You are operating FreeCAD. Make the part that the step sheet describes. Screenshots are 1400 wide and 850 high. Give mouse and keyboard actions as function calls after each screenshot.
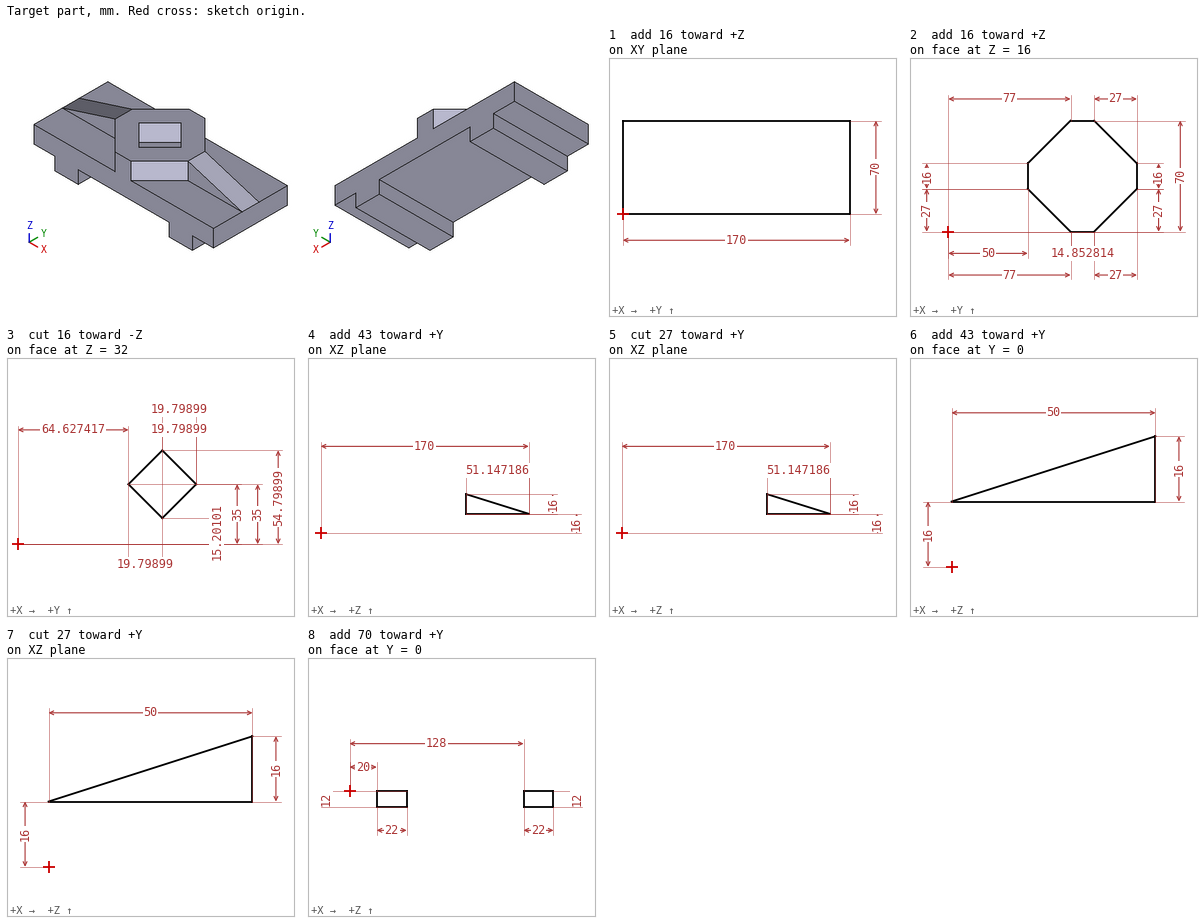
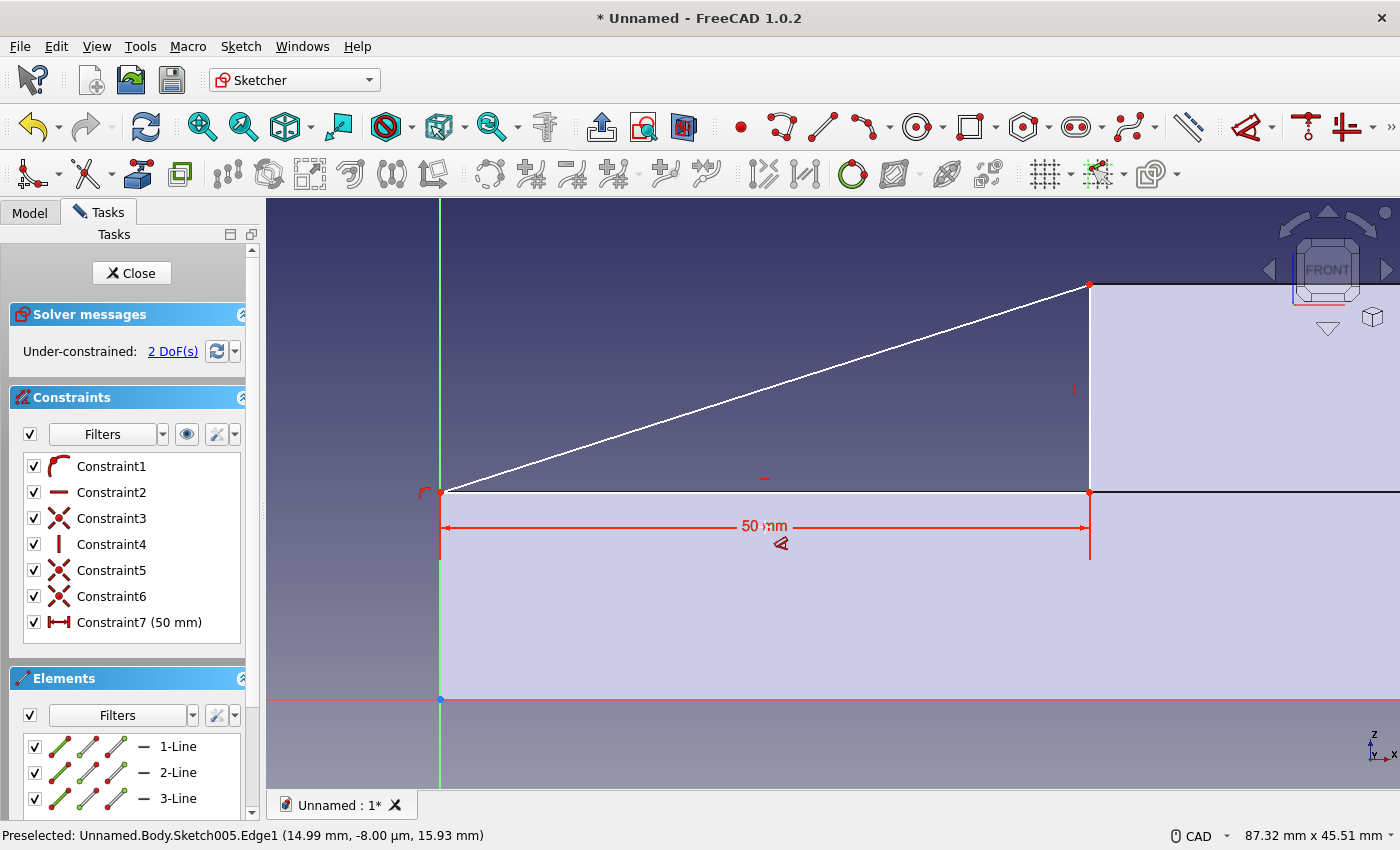
click(1090, 431)
click(1124, 389)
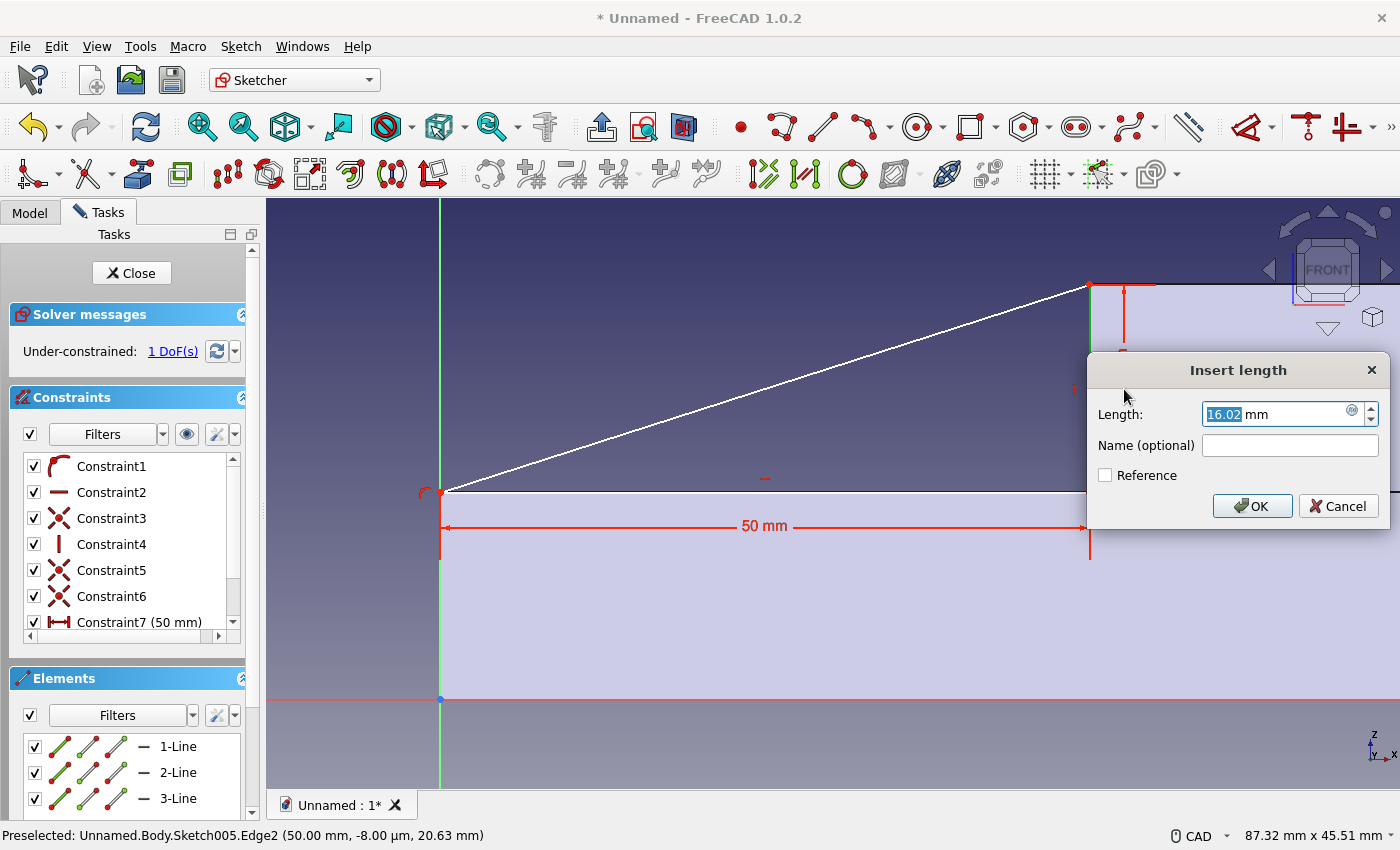
text(16)
key(Return)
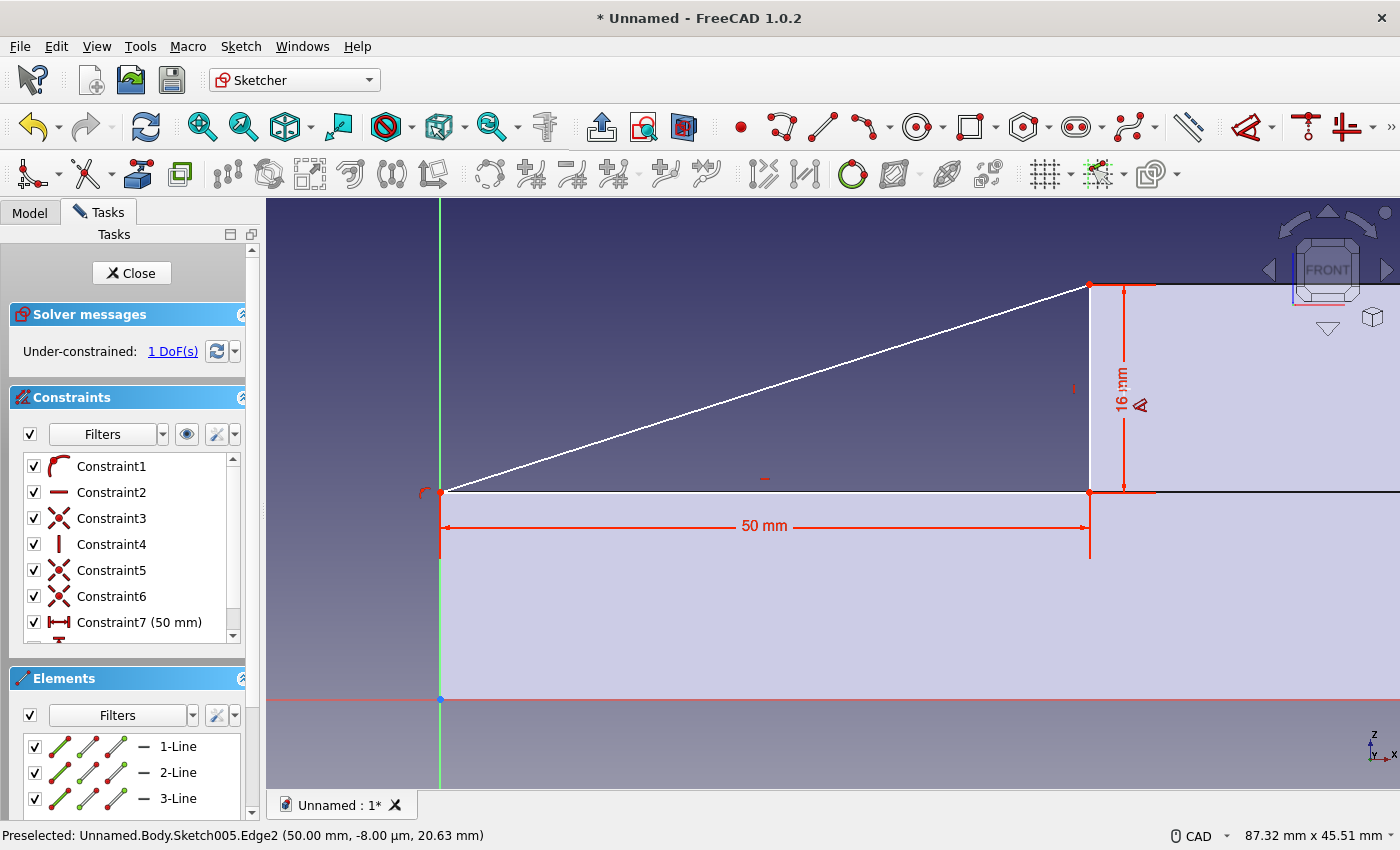
click(440, 493)
click(406, 596)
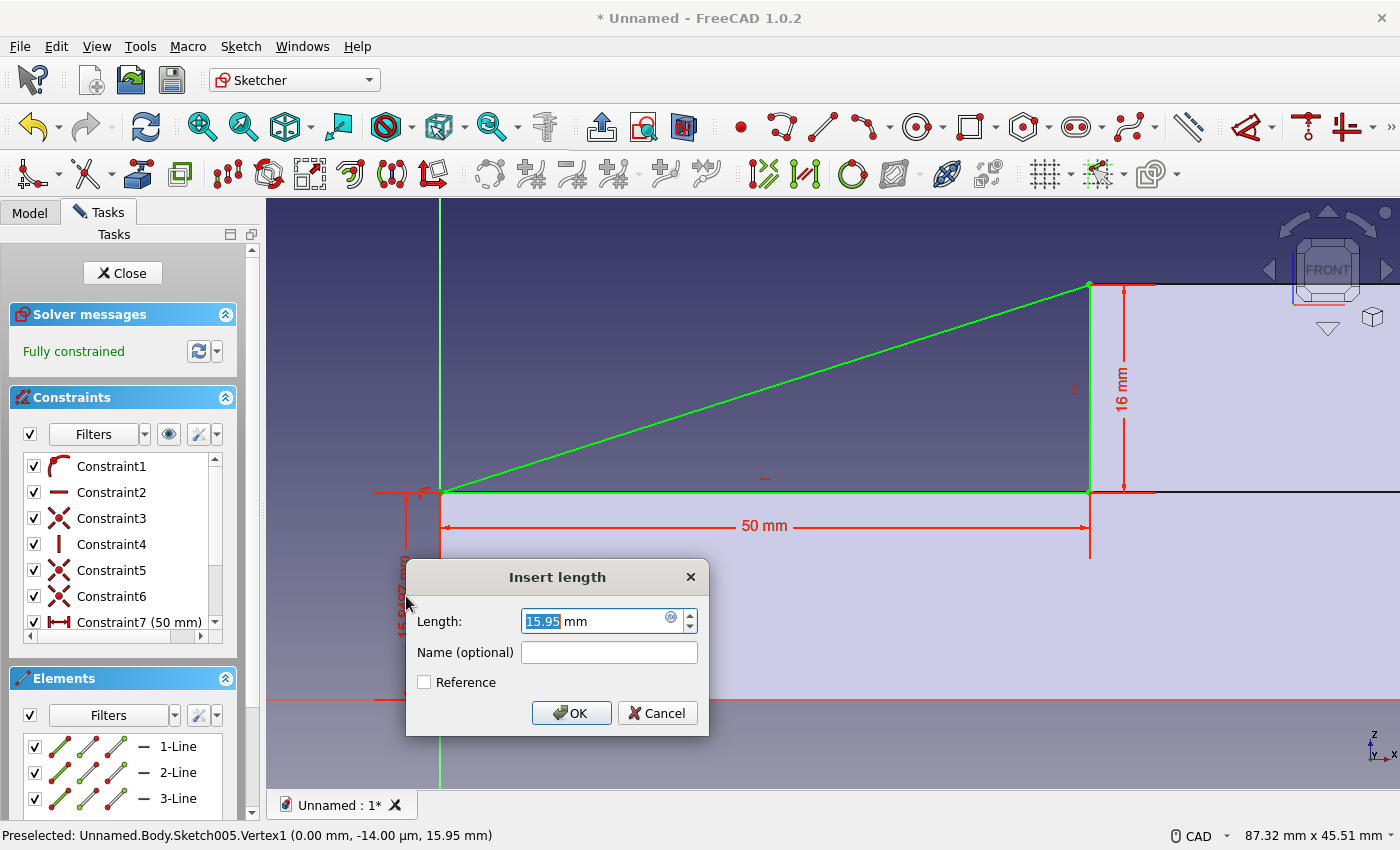
text(16)
key(Return)
key(Escape)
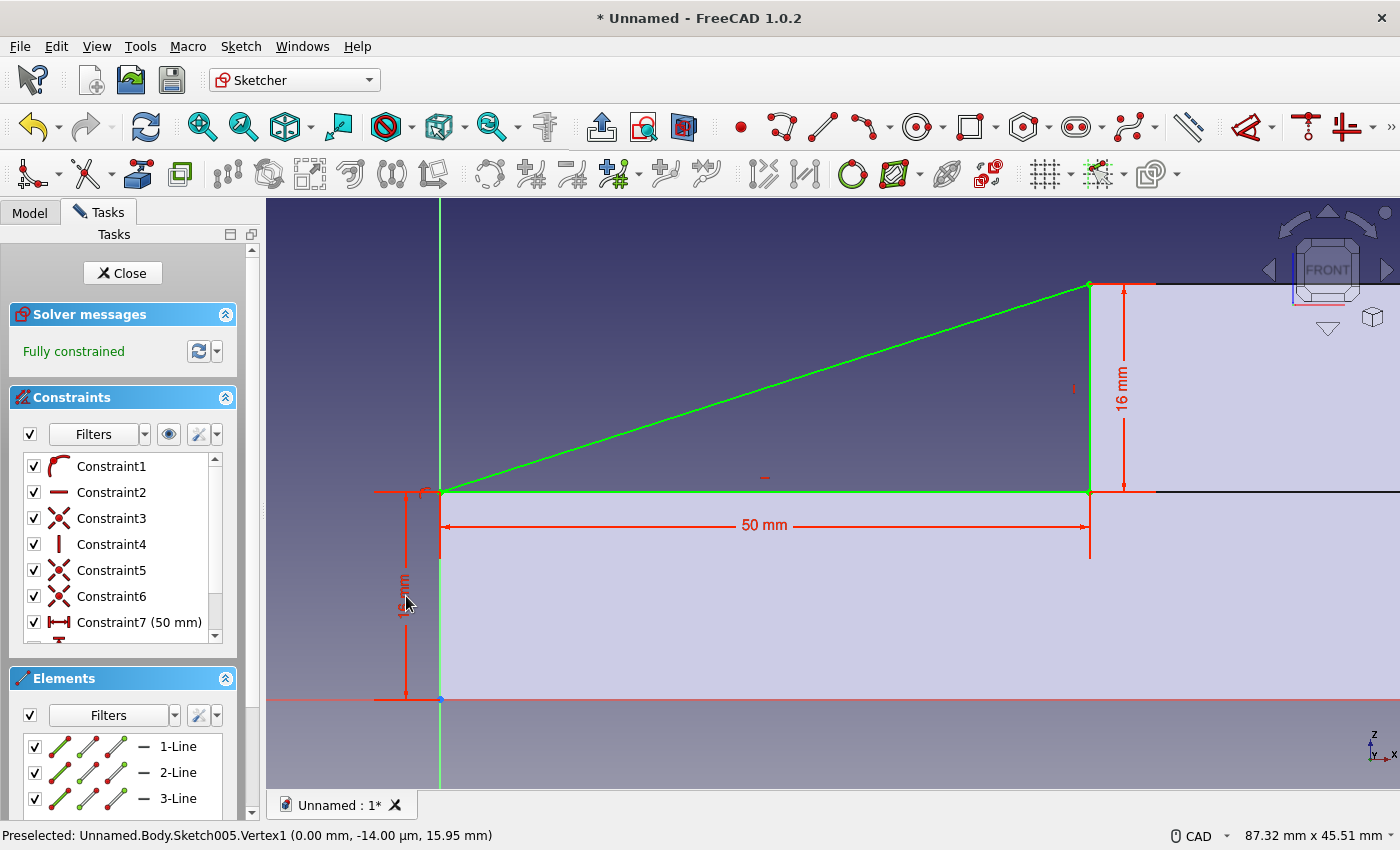
click(123, 273)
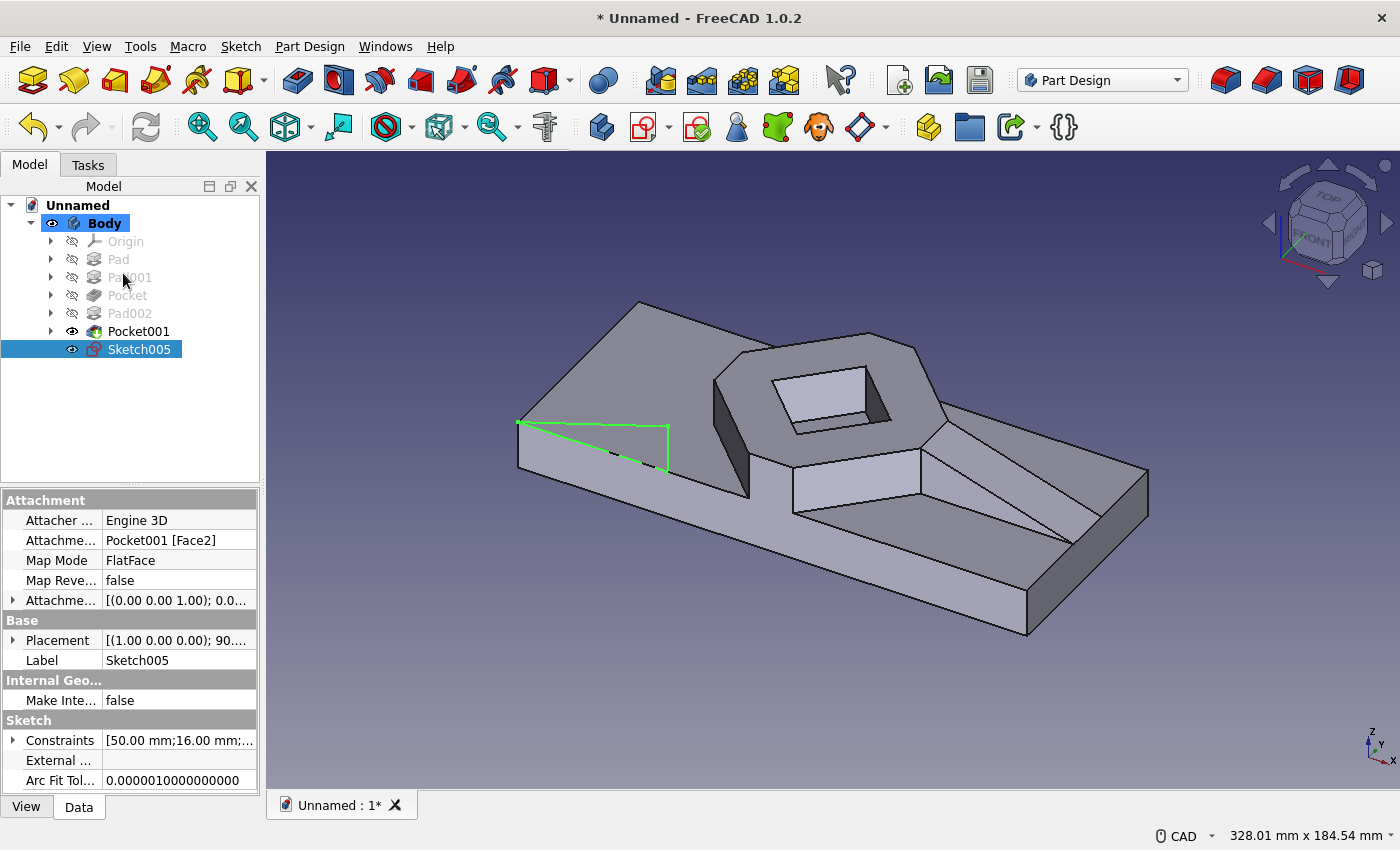
click(33, 80)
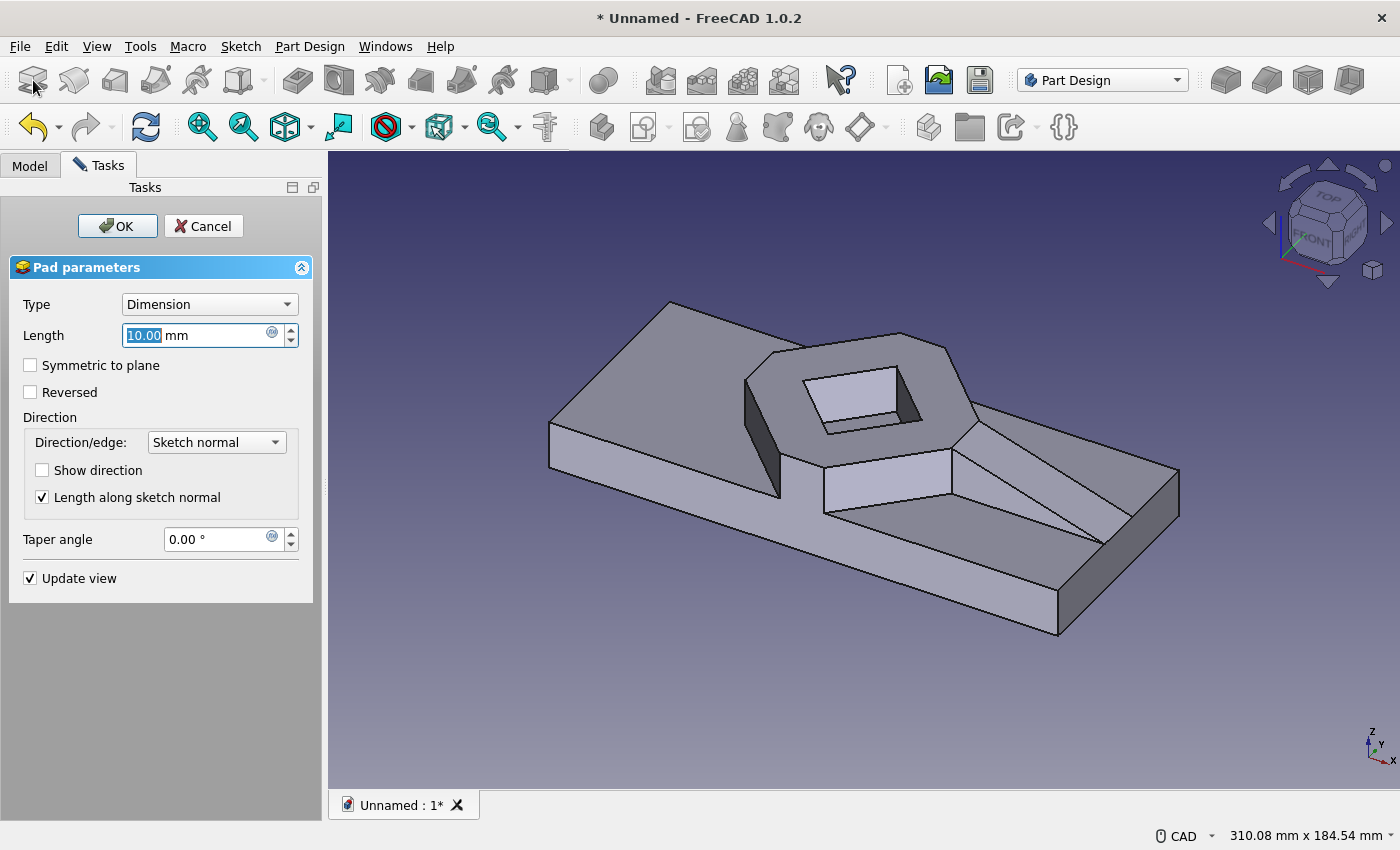
text(43)
key(Tab)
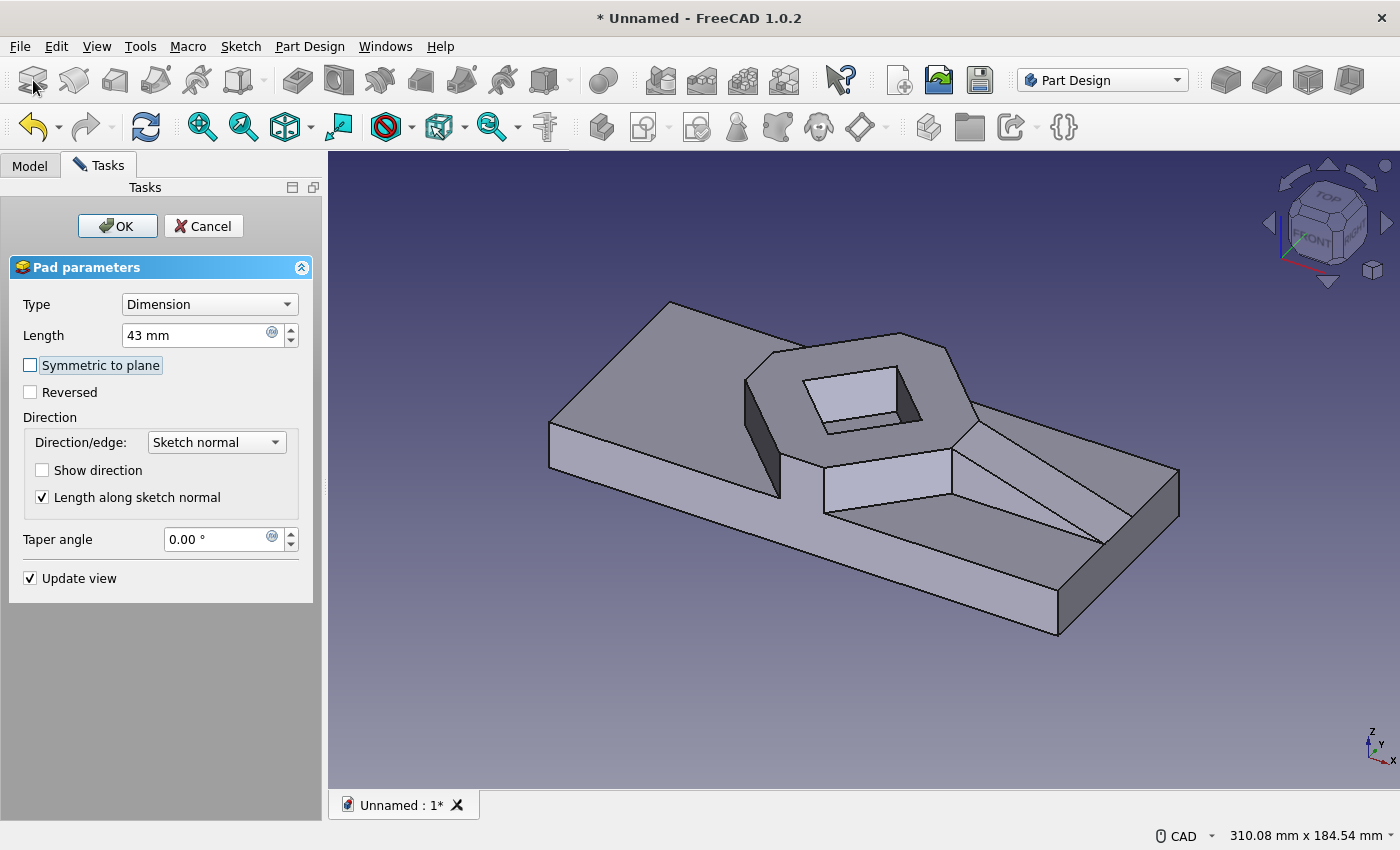
click(31, 392)